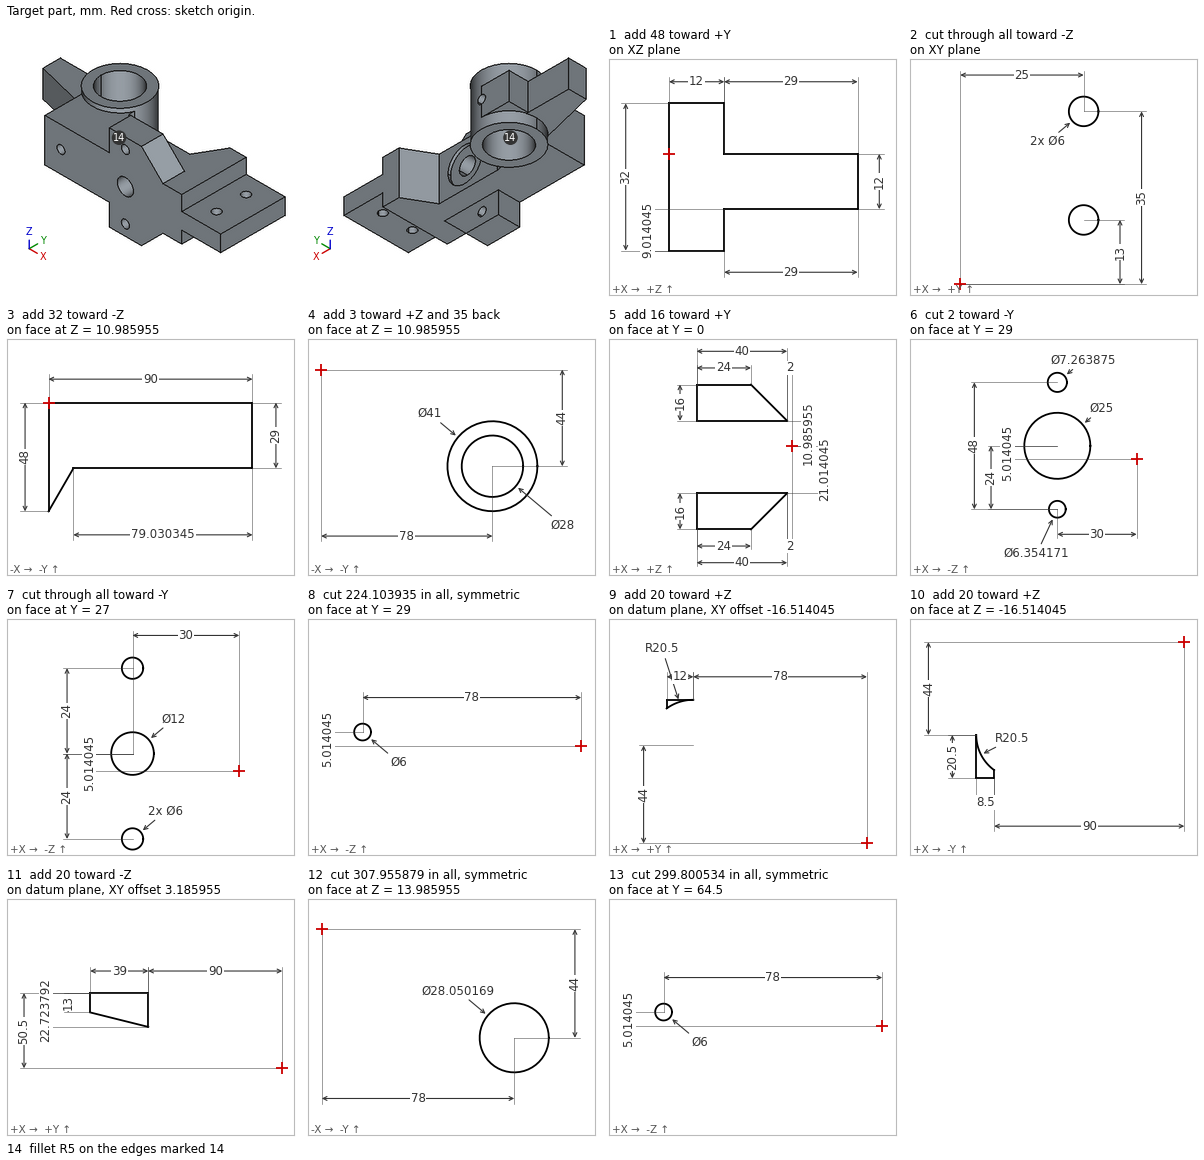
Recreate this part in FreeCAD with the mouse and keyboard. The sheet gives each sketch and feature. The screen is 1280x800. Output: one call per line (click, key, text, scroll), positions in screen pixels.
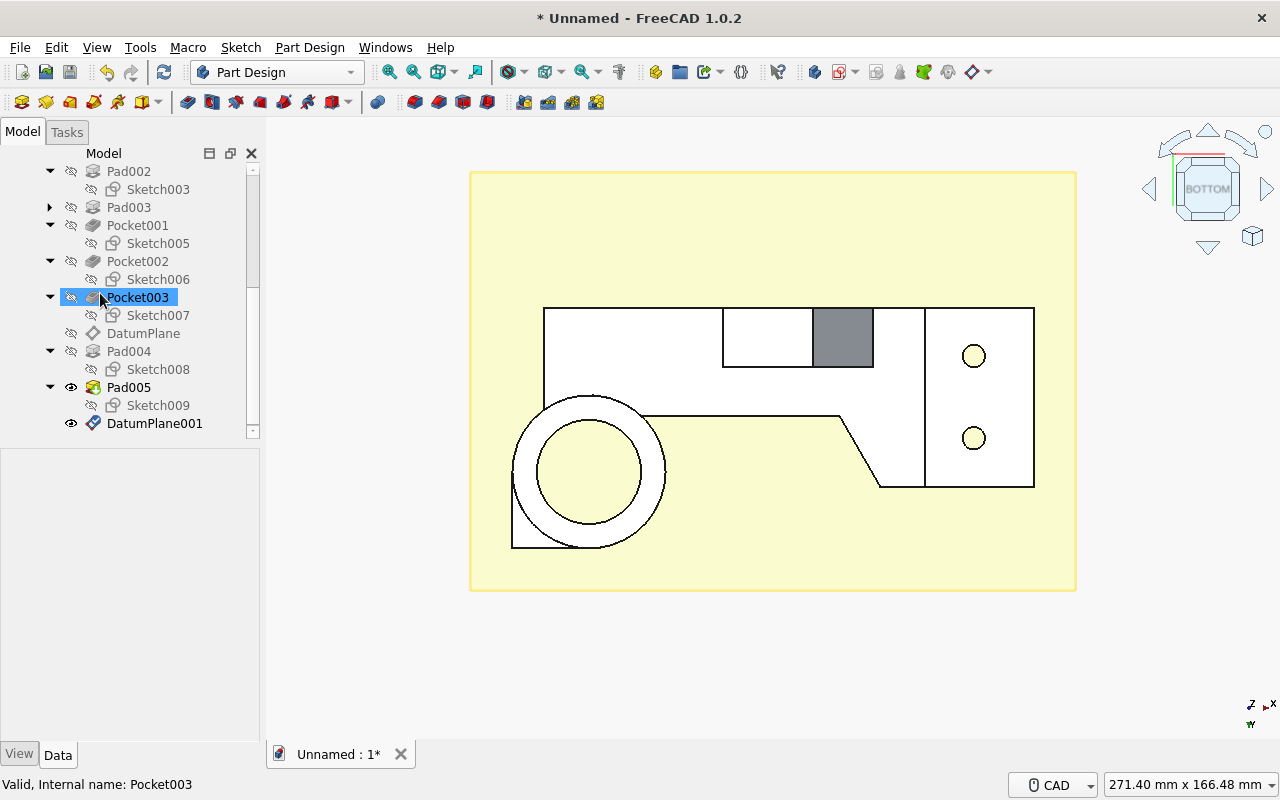
click(116, 423)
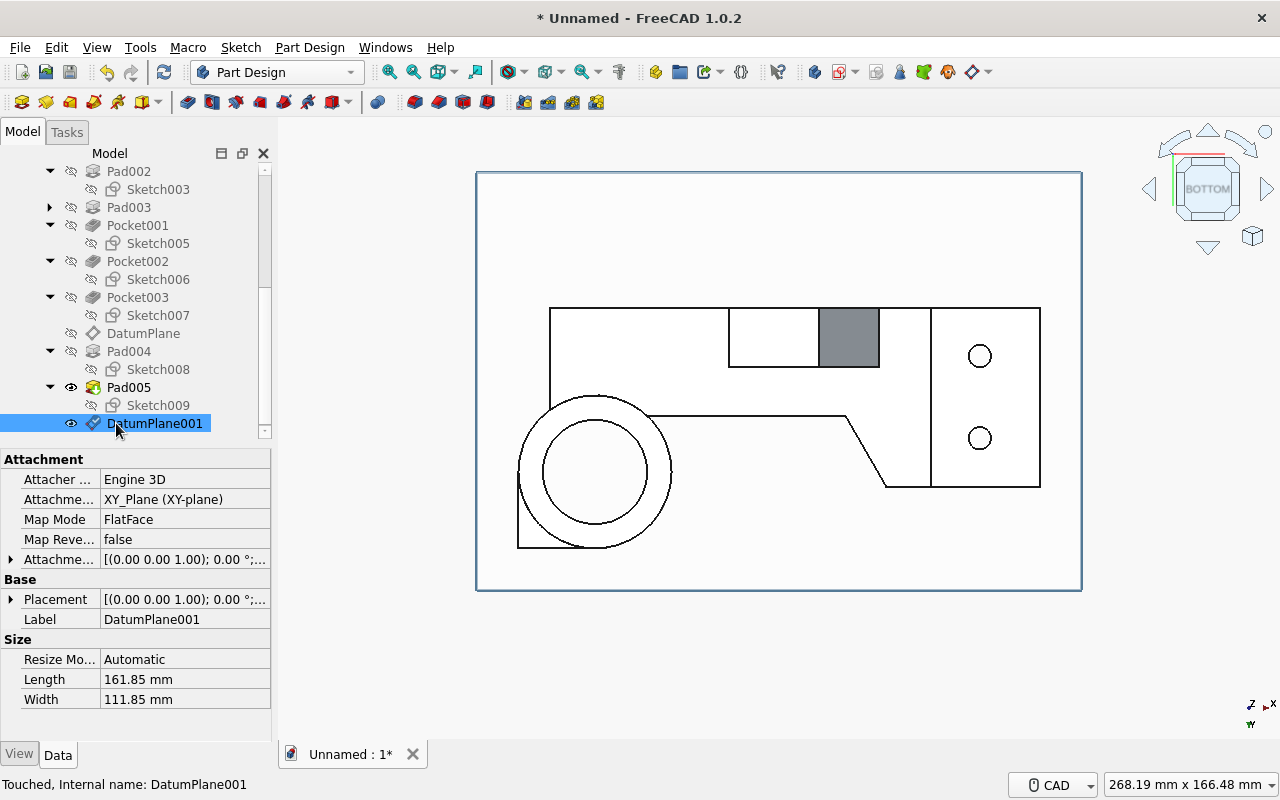
click(840, 72)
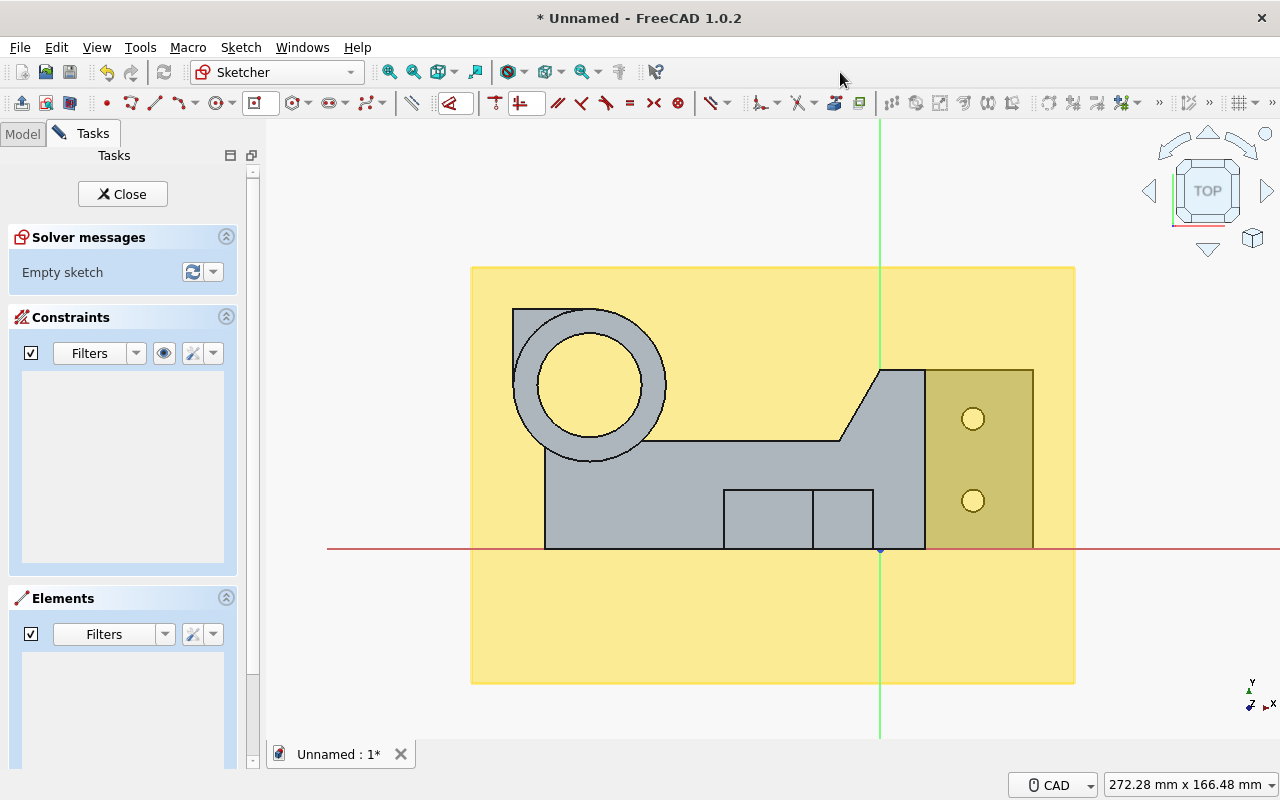
key(q)
key(s)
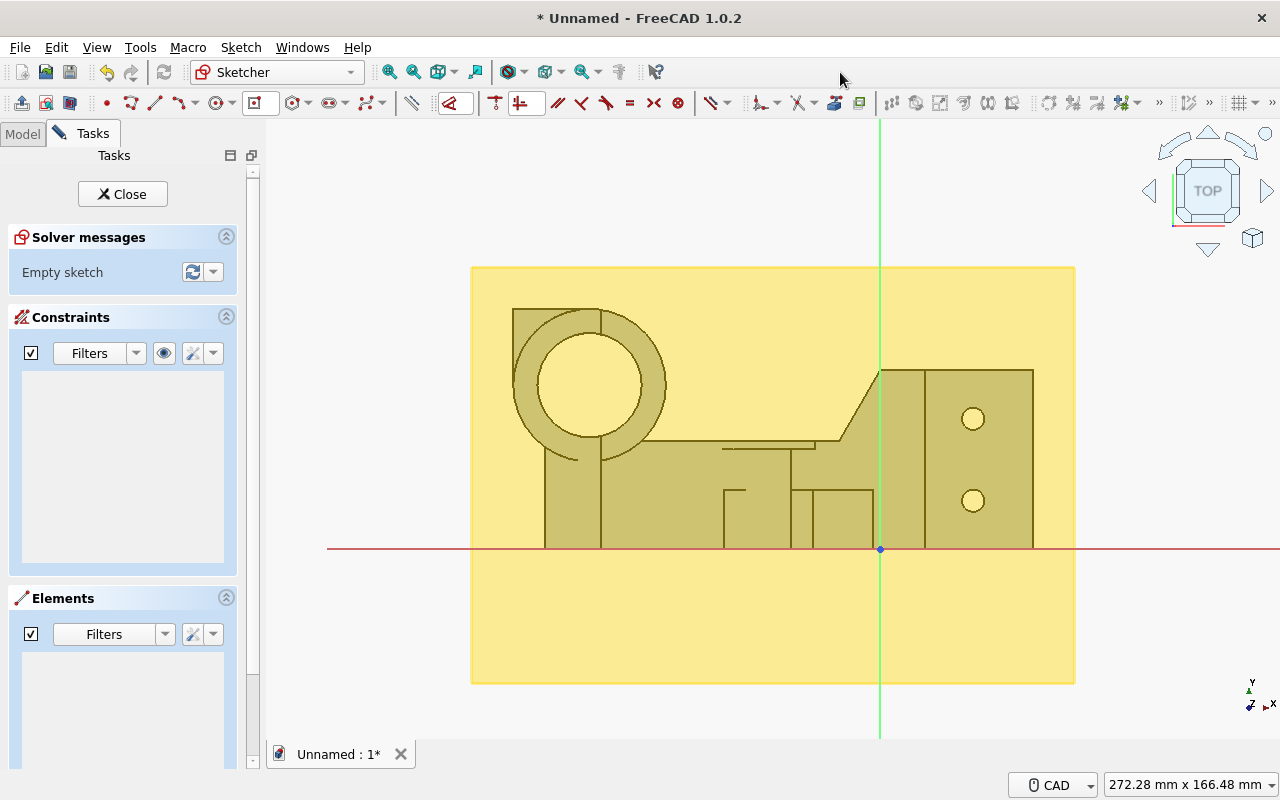
scroll(396, 395, up, 7)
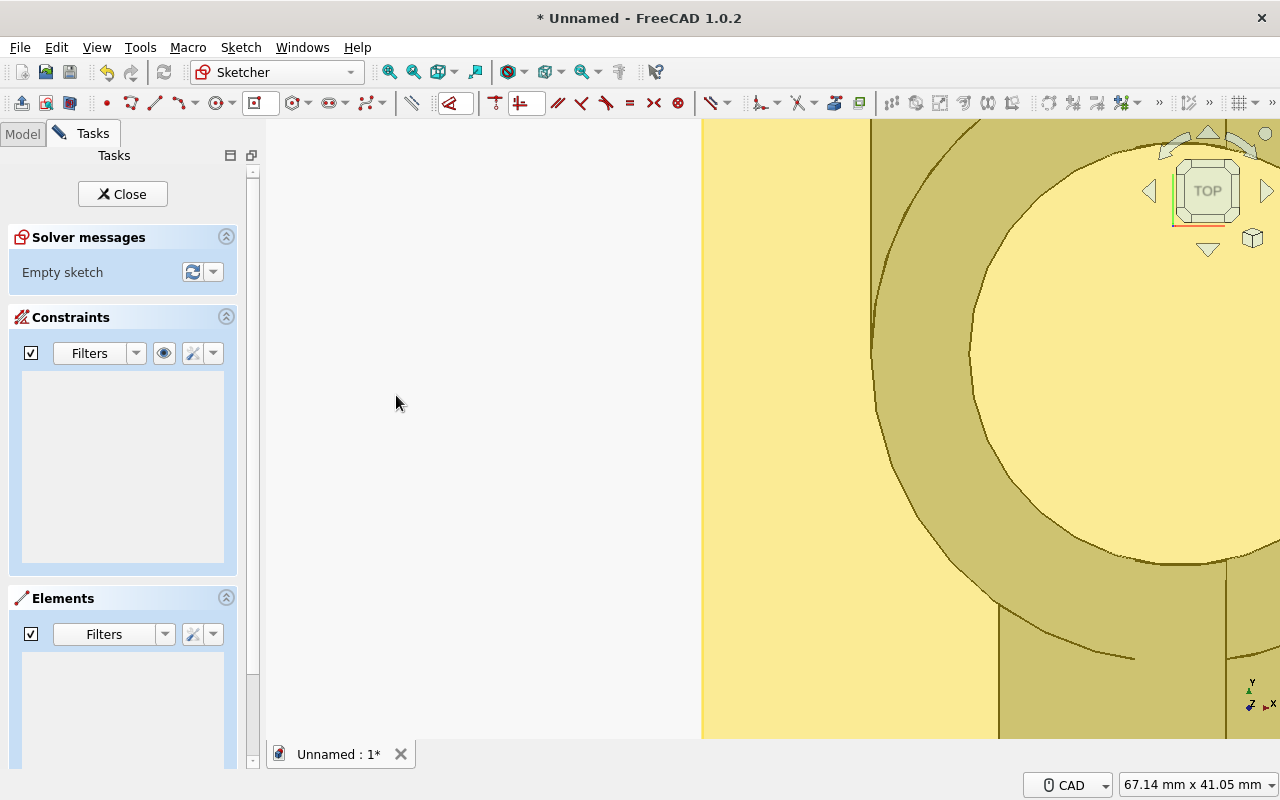
click(132, 104)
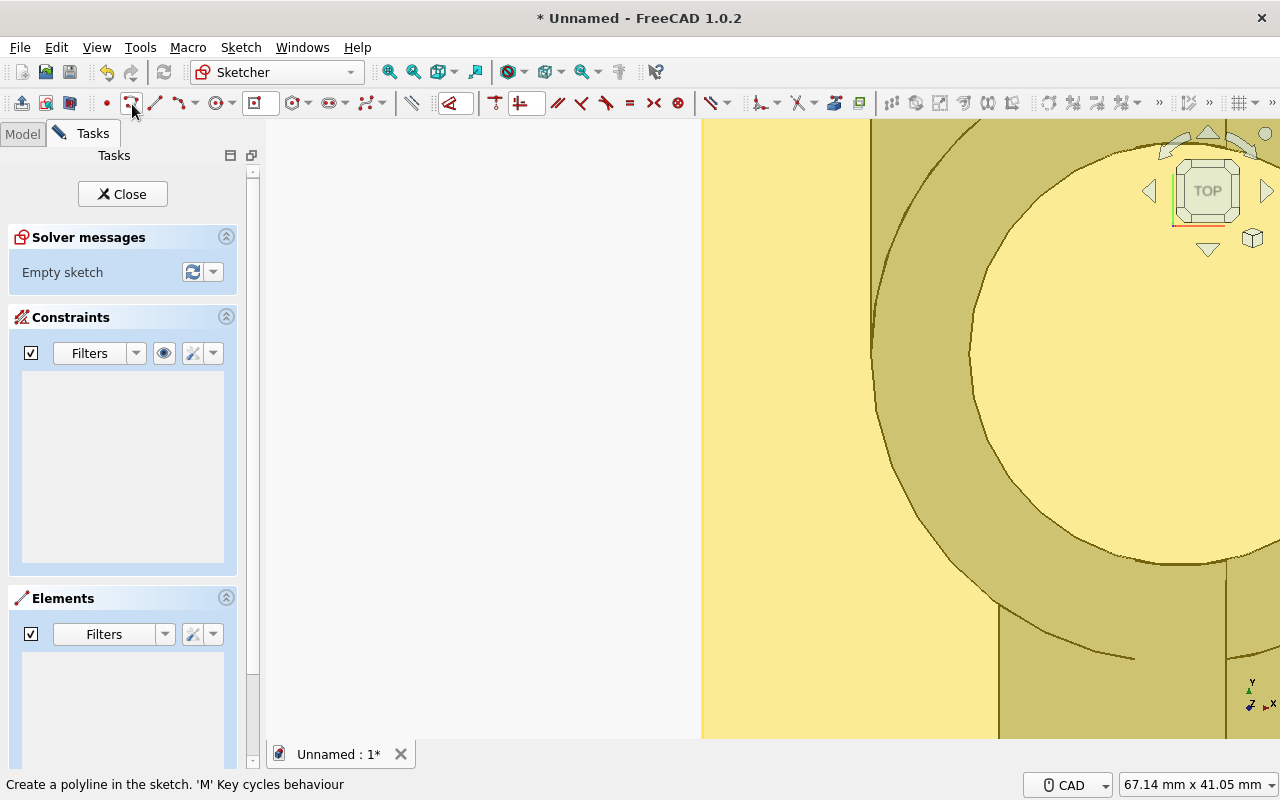
click(999, 599)
click(999, 256)
click(410, 256)
click(410, 452)
click(999, 600)
key(Escape)
key(Escape)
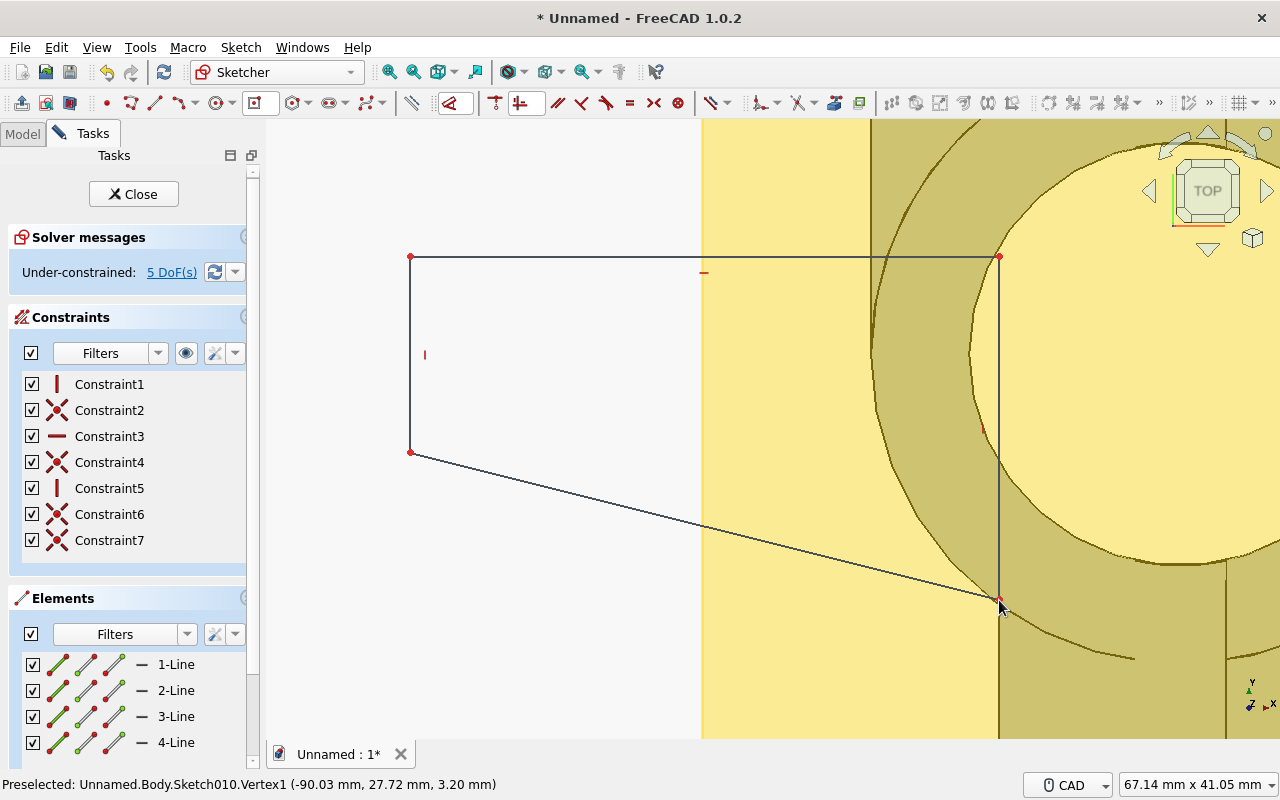
click(822, 257)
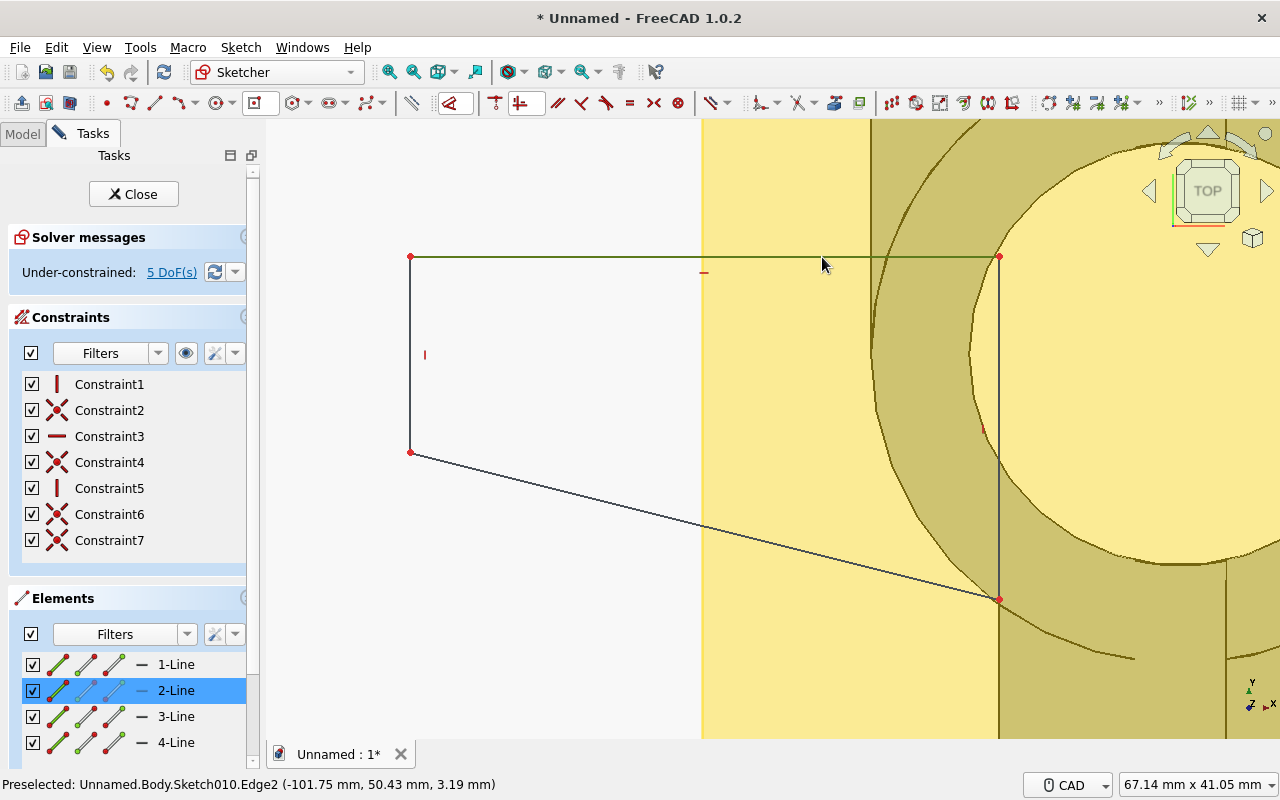
key(l)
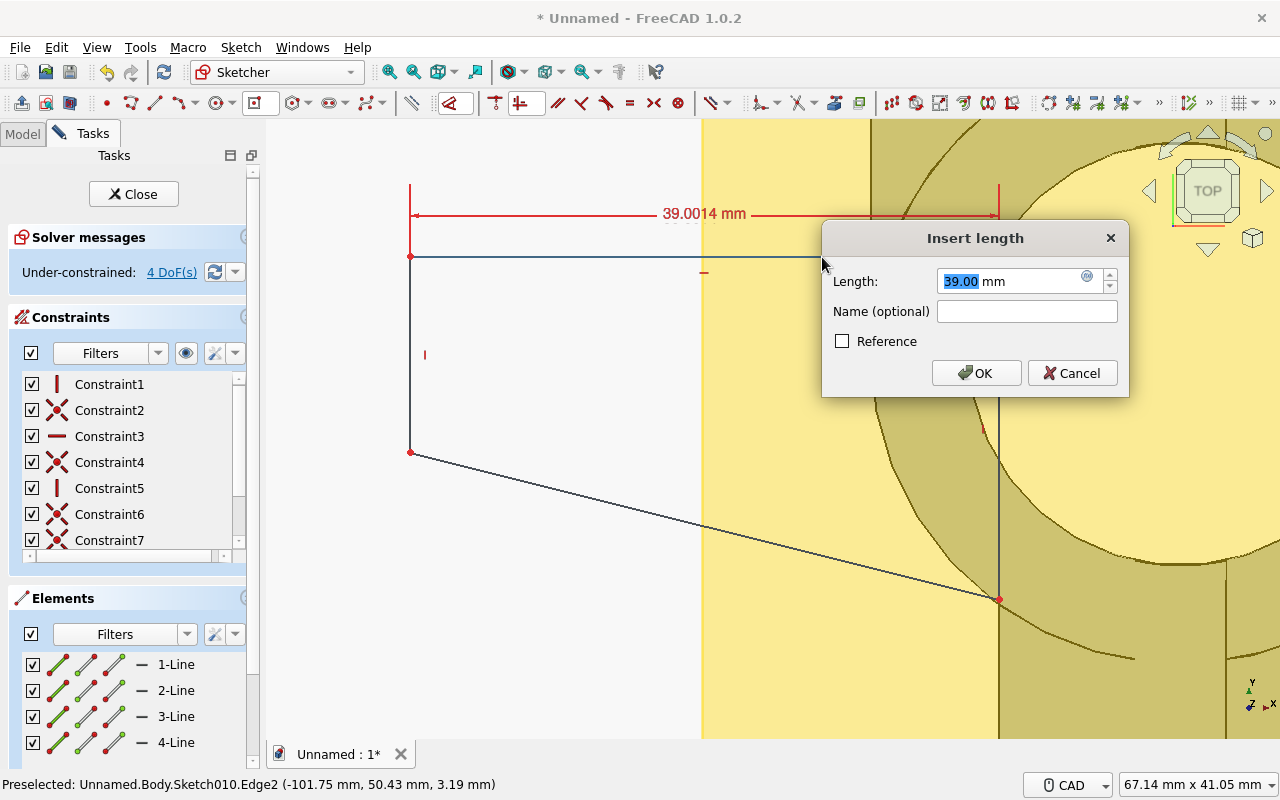
text(39)
key(Return)